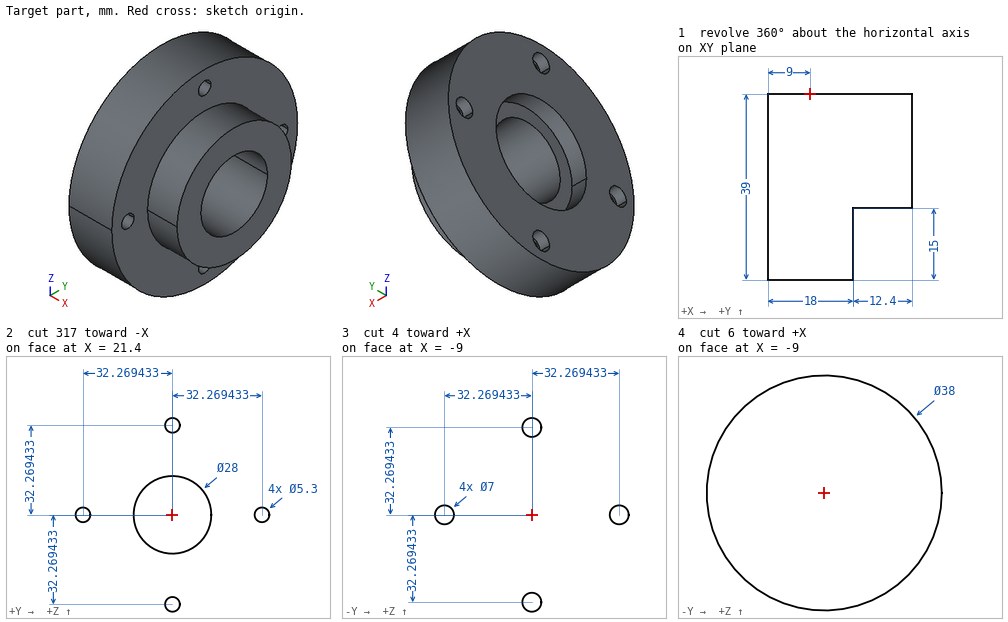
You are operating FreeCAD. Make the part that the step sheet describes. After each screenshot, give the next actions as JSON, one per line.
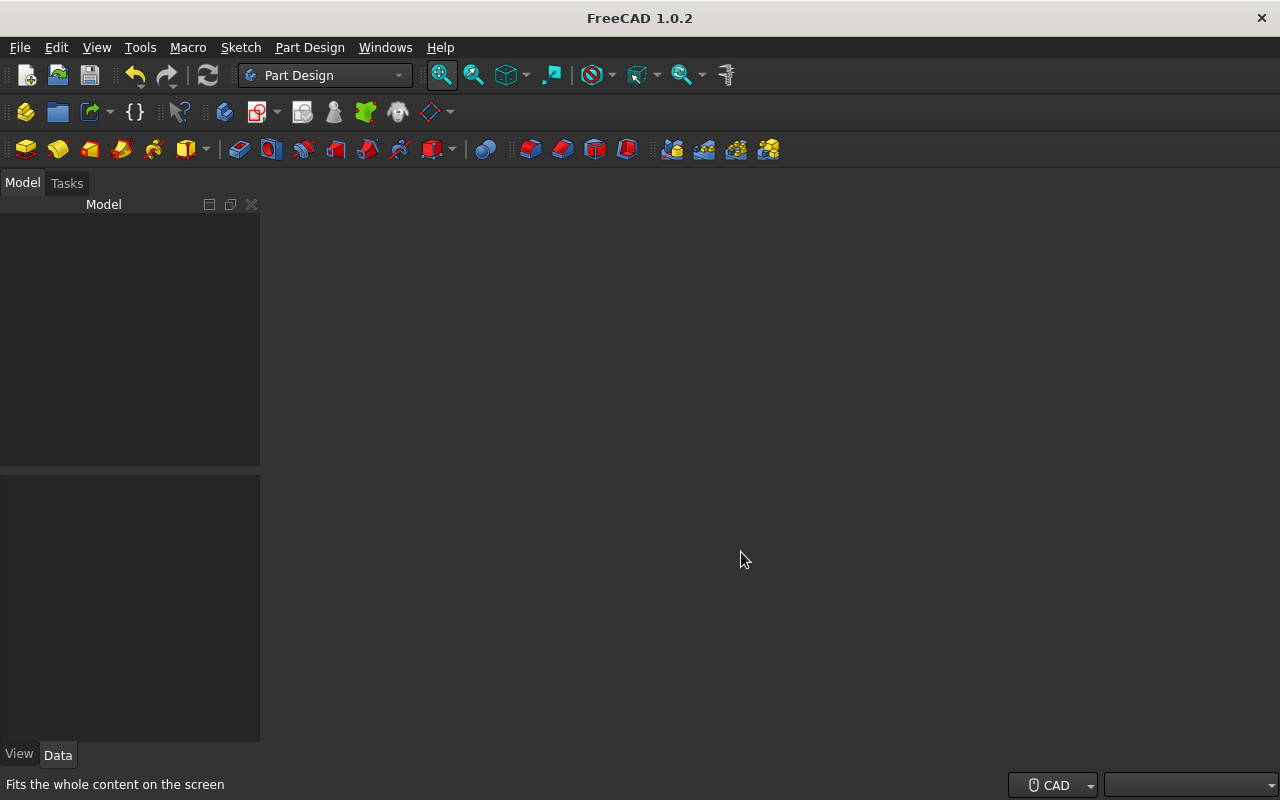
{"action": "left_click", "coordinate": [26, 76]}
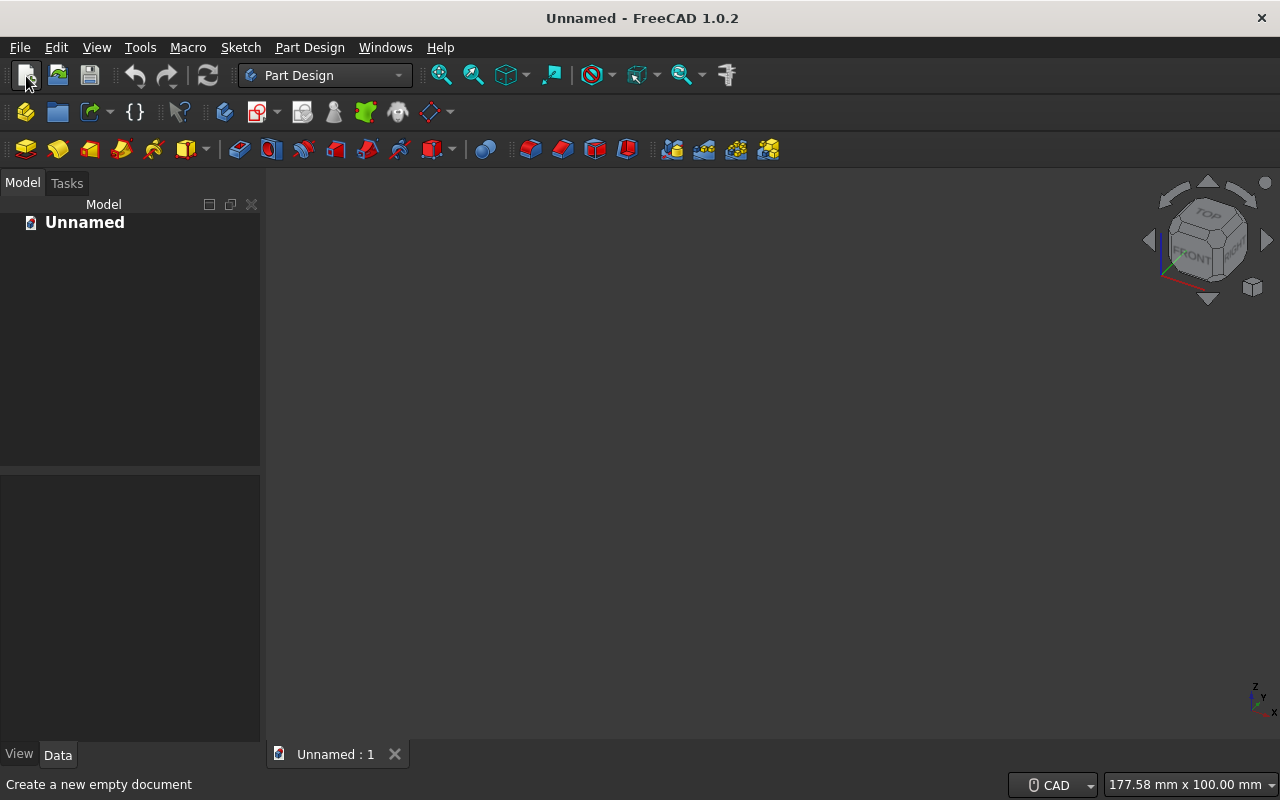
{"action": "left_click", "coordinate": [258, 112]}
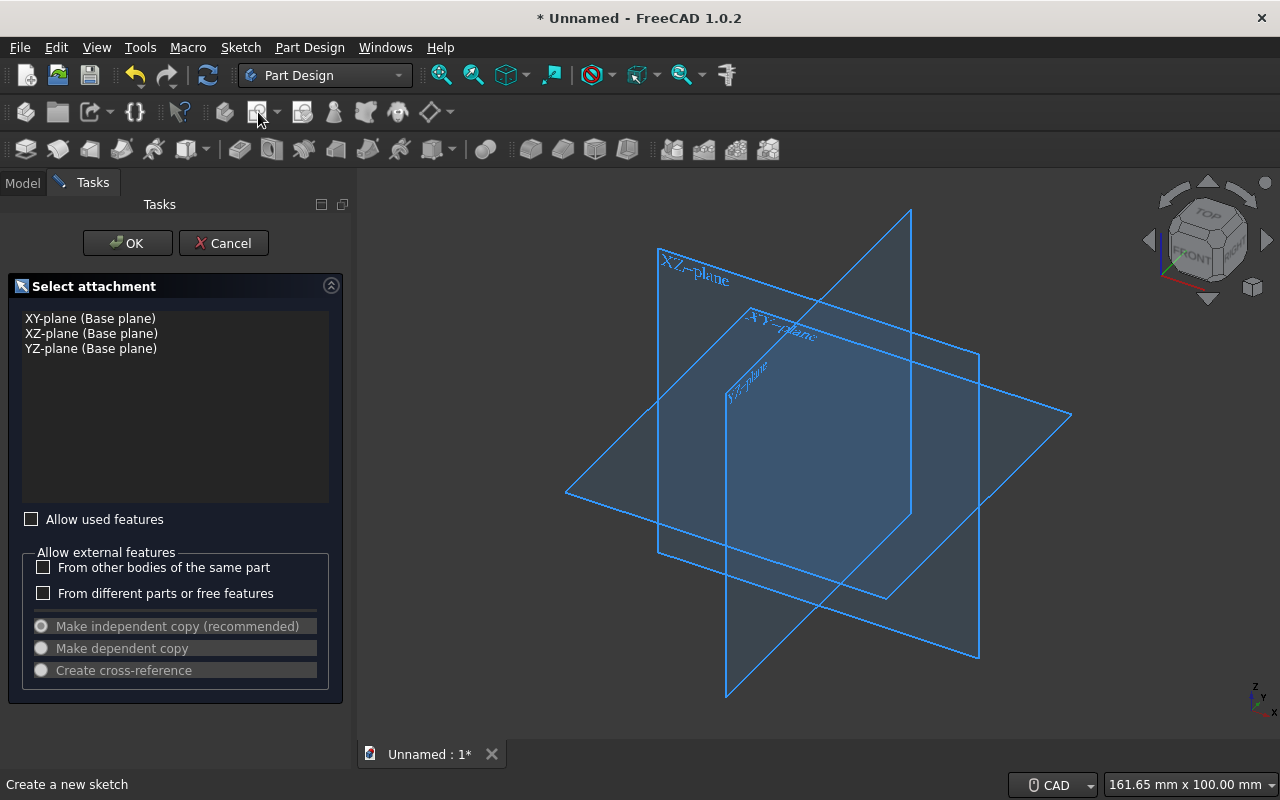
{"action": "left_click", "coordinate": [82, 318]}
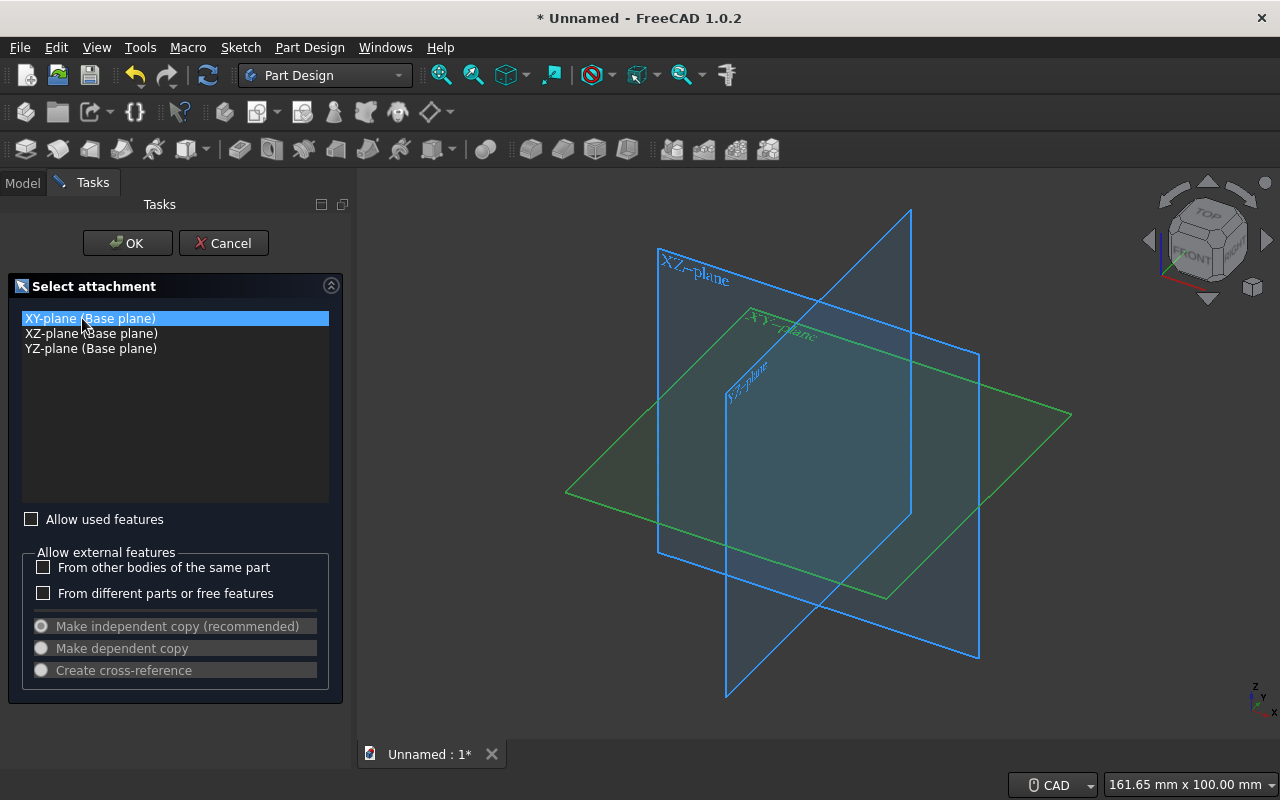
{"action": "left_click", "coordinate": [128, 243]}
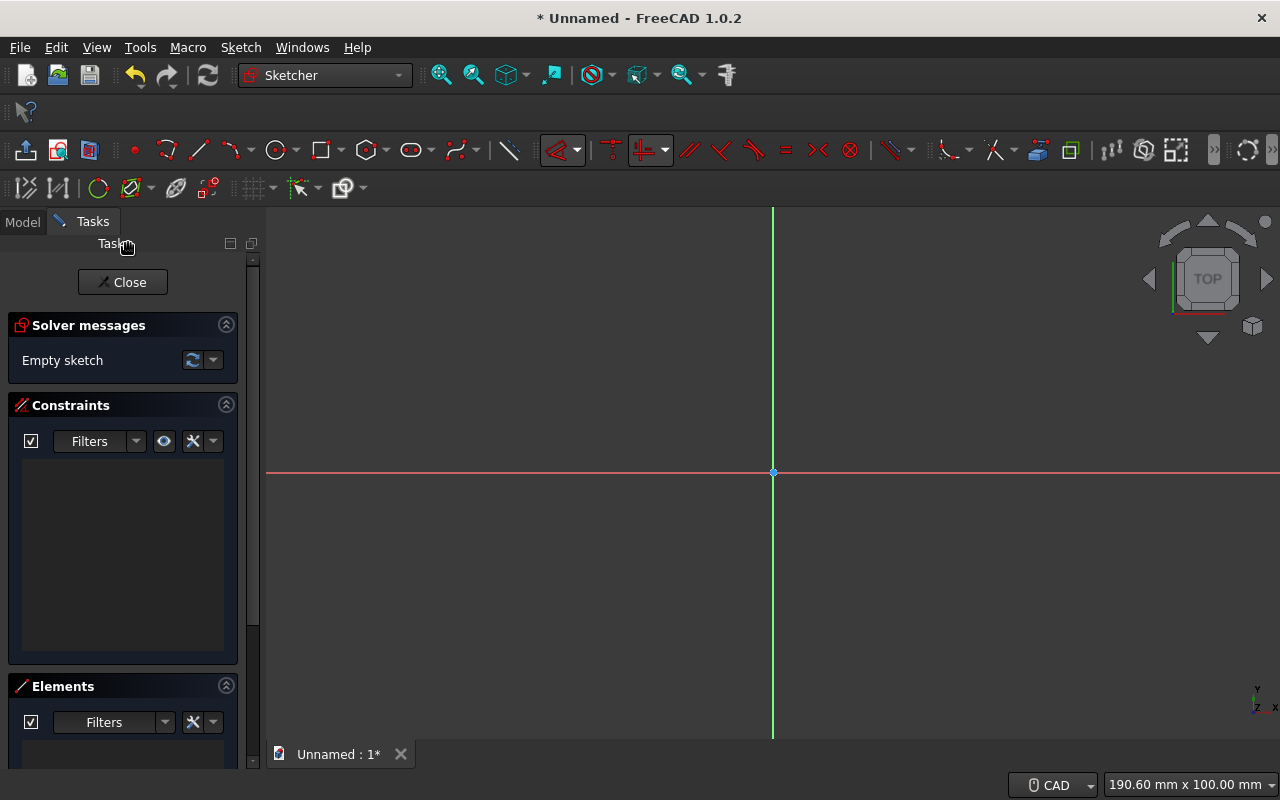
{"action": "scroll", "coordinate": [1012, 711], "scroll_direction": "up", "scroll_amount": 2}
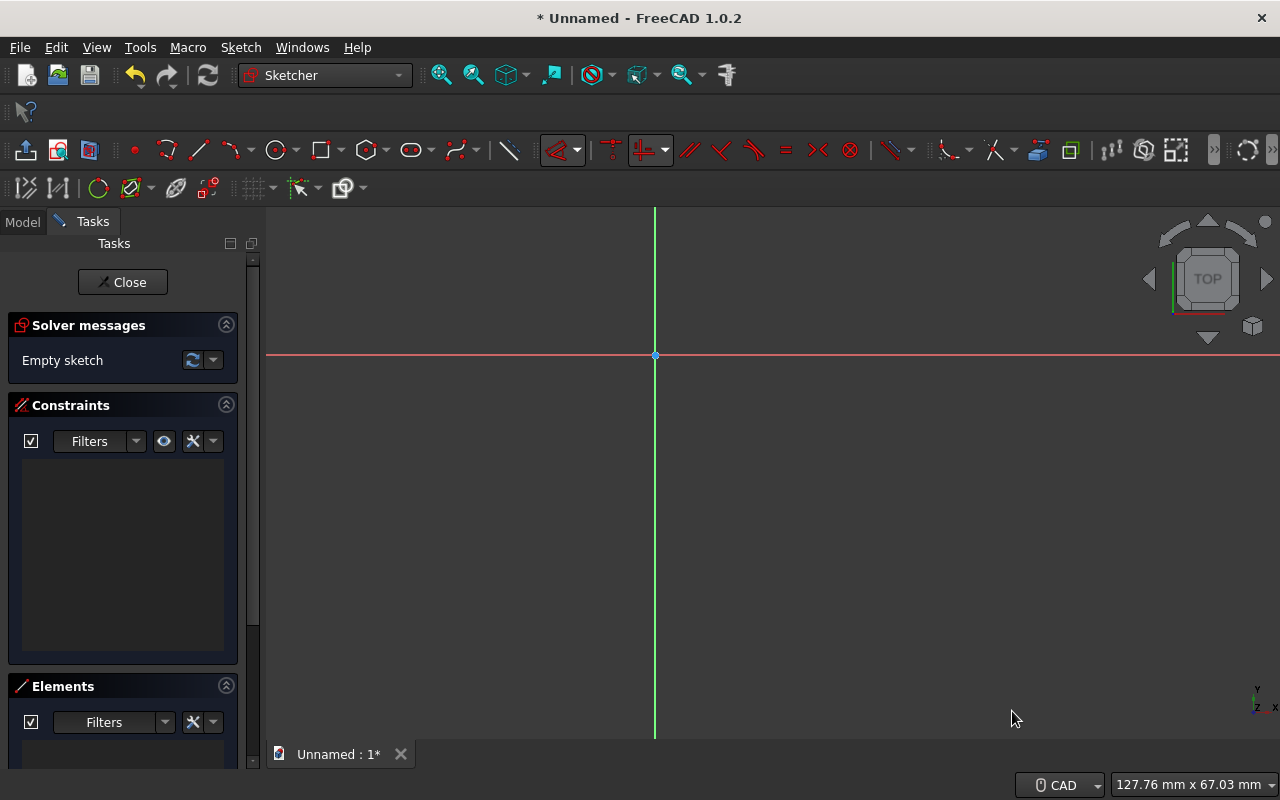
{"action": "left_click", "coordinate": [168, 150]}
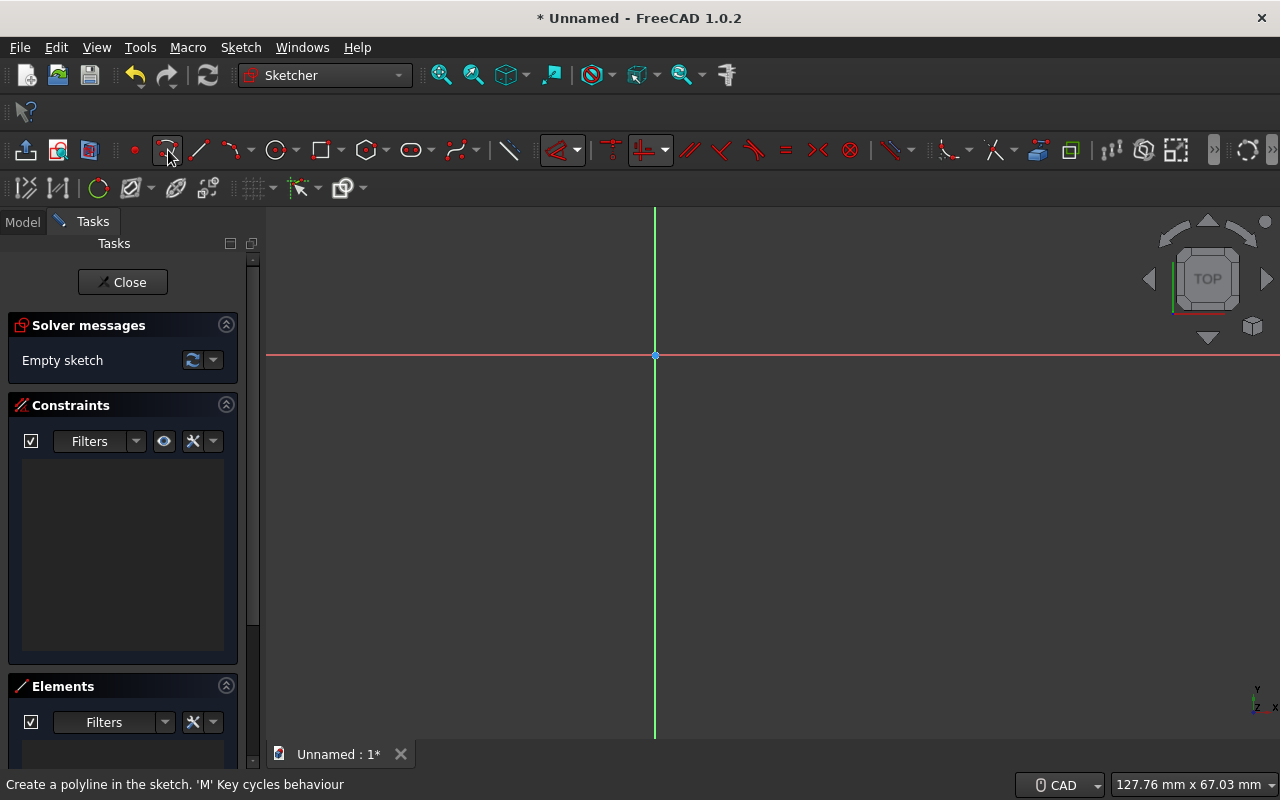
{"action": "left_click", "coordinate": [584, 355]}
{"action": "left_click", "coordinate": [584, 665]}
{"action": "left_click", "coordinate": [727, 665]}
{"action": "left_click", "coordinate": [727, 546]}
{"action": "left_click", "coordinate": [825, 546]}
{"action": "left_click", "coordinate": [825, 364]}
{"action": "left_click", "coordinate": [584, 355]}
{"action": "key", "text": "Escape"}
{"action": "key", "text": "Escape"}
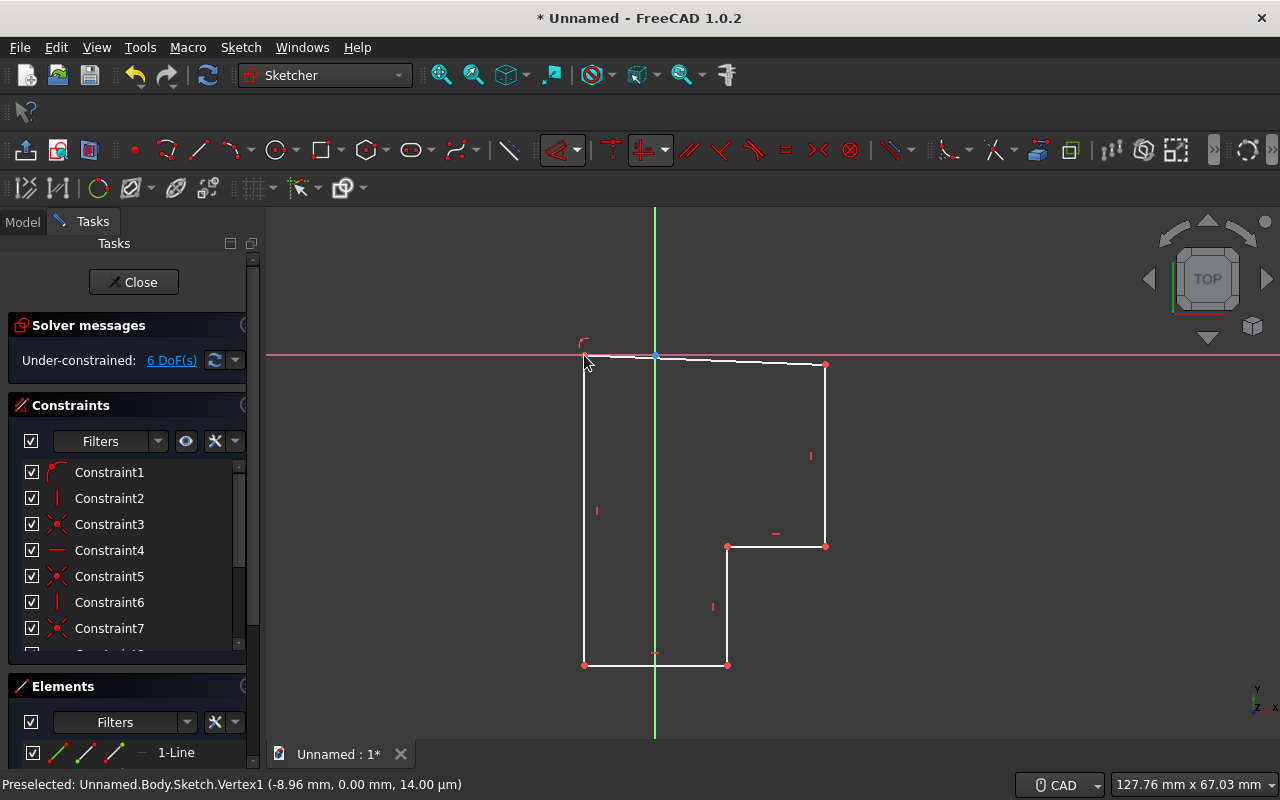
{"action": "left_click", "coordinate": [680, 359]}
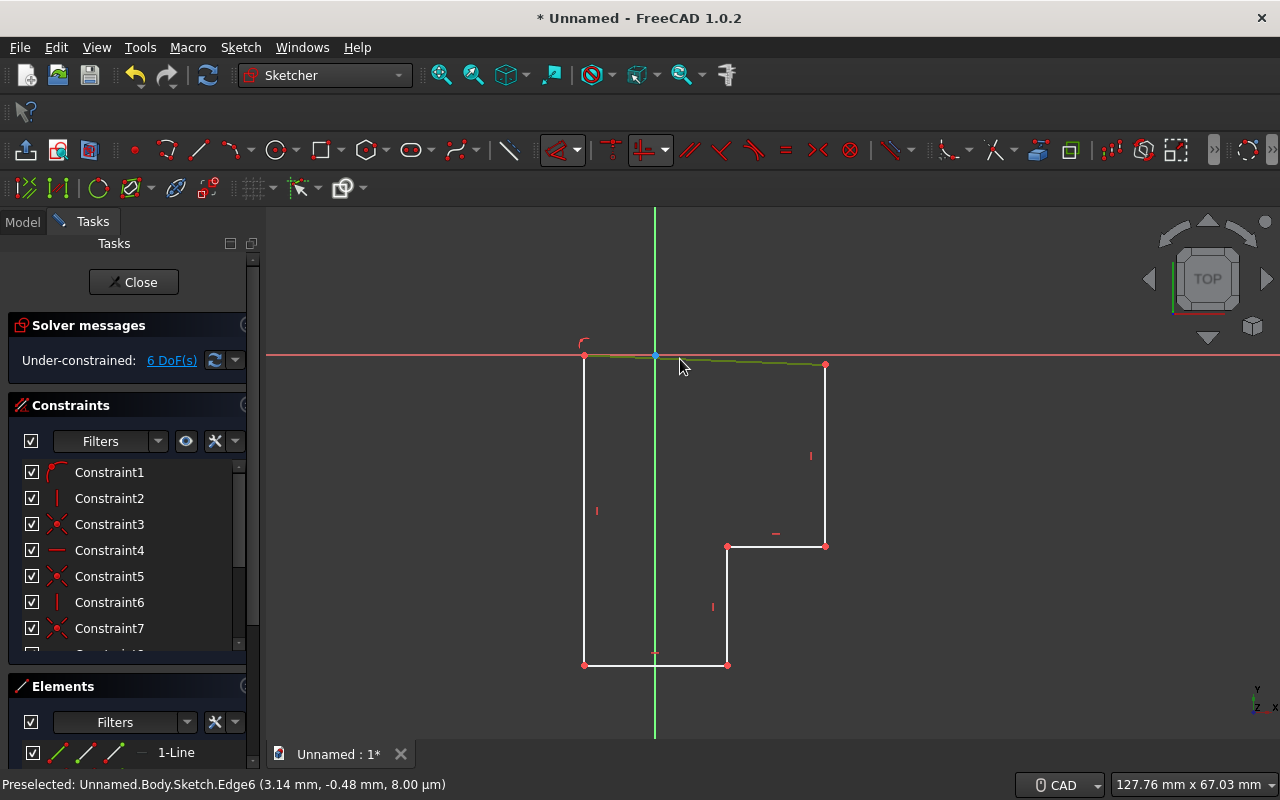
{"action": "key", "text": "h"}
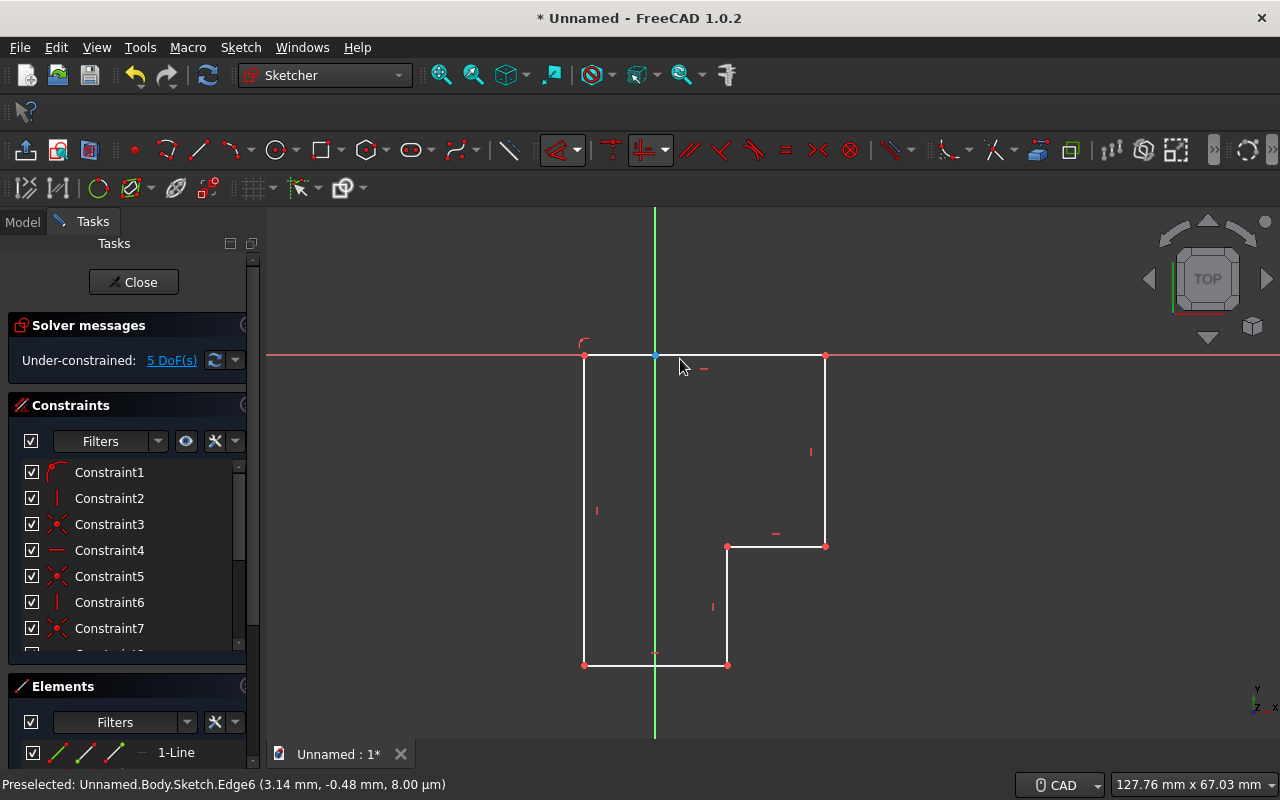
{"action": "left_click", "coordinate": [584, 449]}